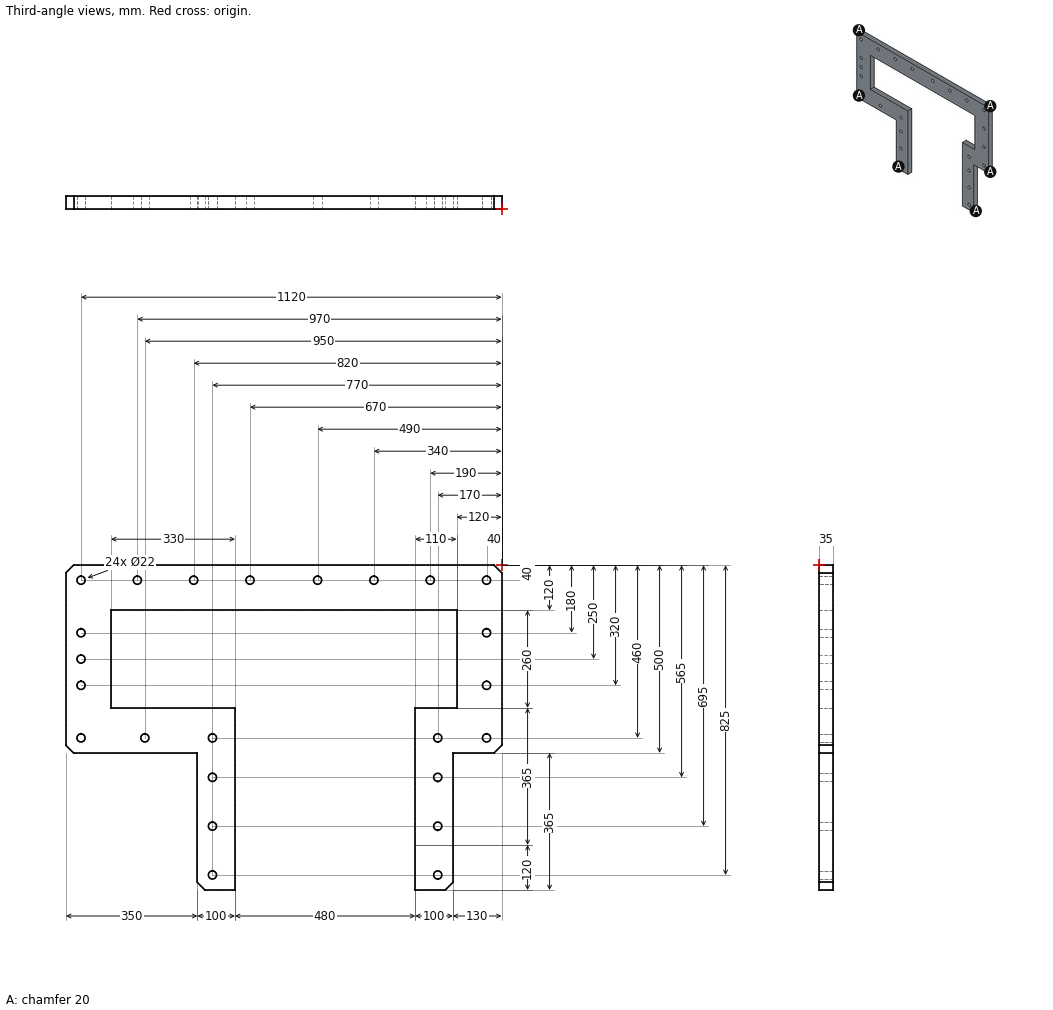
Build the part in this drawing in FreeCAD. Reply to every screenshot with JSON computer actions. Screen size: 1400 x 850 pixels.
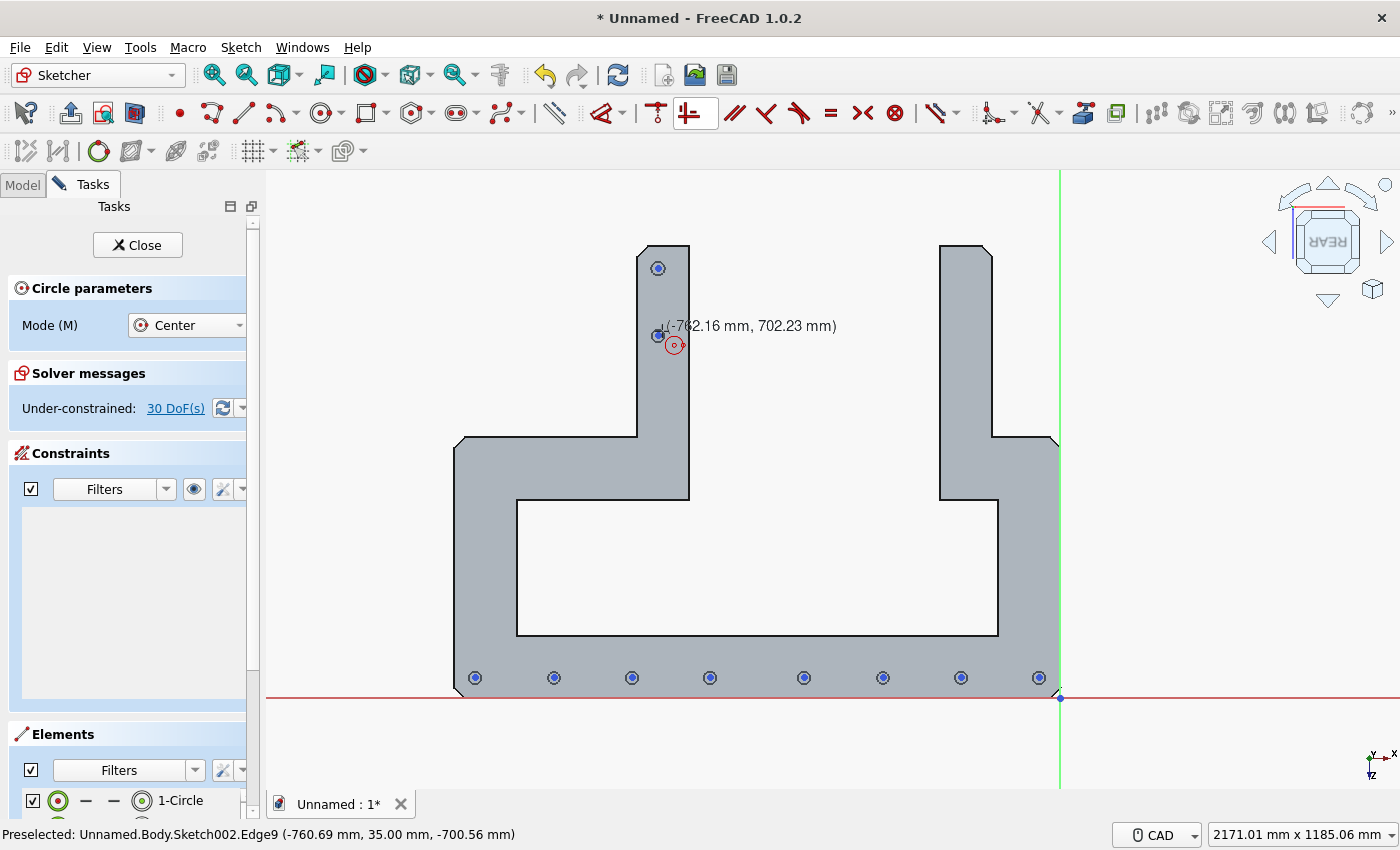
{"action": "left_click", "coordinate": [658, 403]}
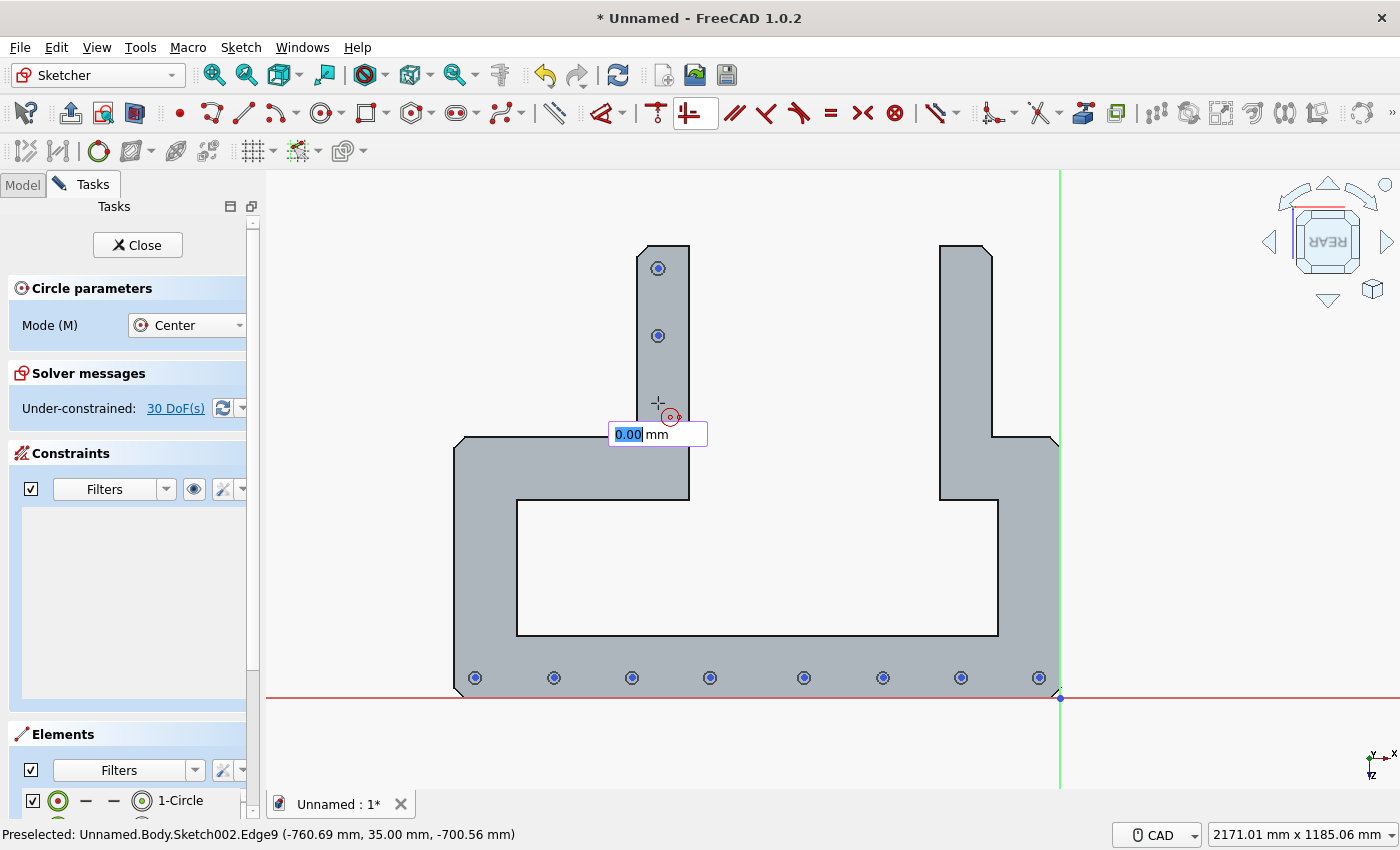
{"action": "scroll", "coordinate": [662, 399], "scroll_direction": "up", "scroll_amount": 6}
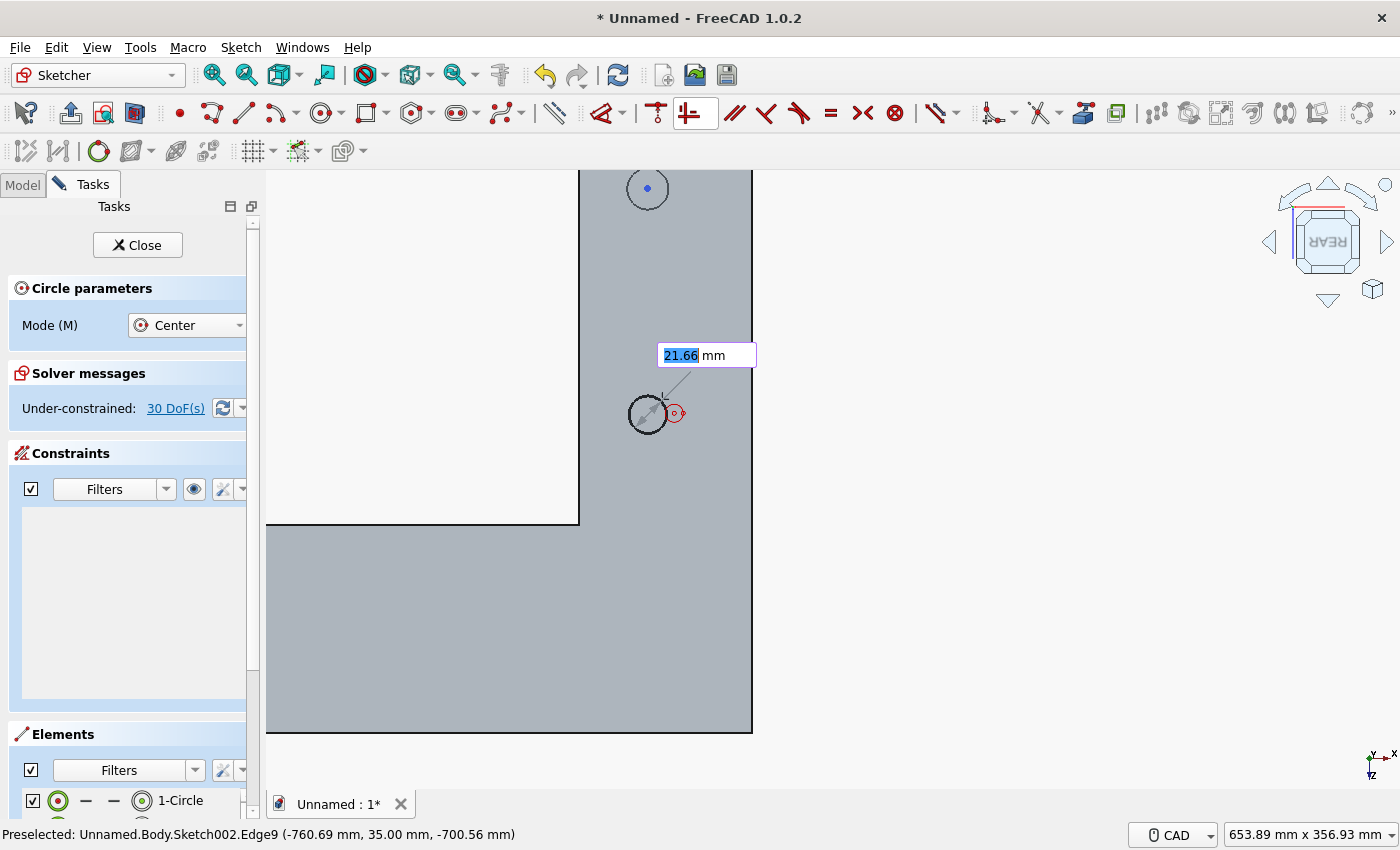
{"action": "left_click", "coordinate": [662, 398]}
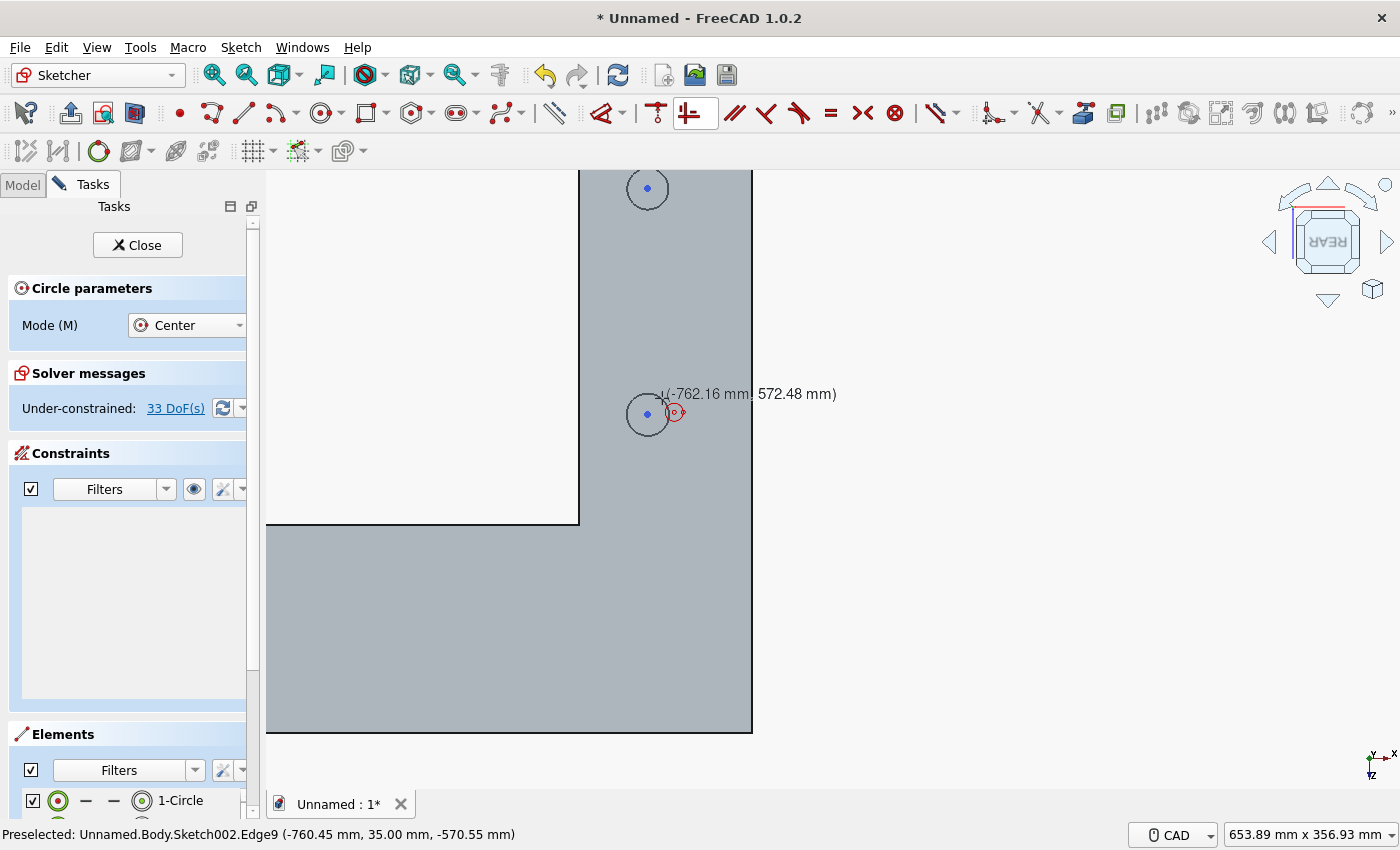
{"action": "scroll", "coordinate": [662, 399], "scroll_direction": "down", "scroll_amount": 6}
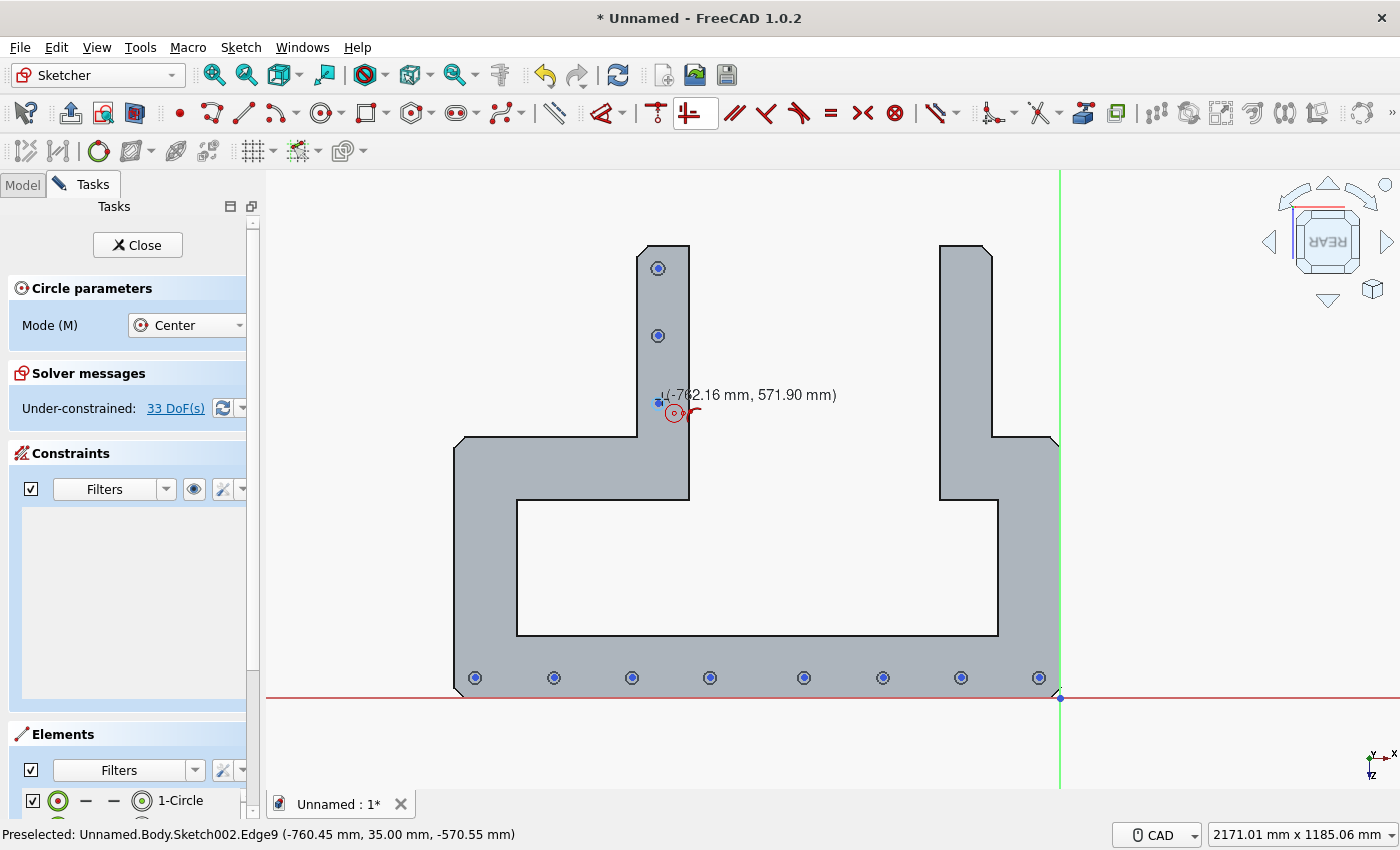
{"action": "left_click", "coordinate": [658, 458]}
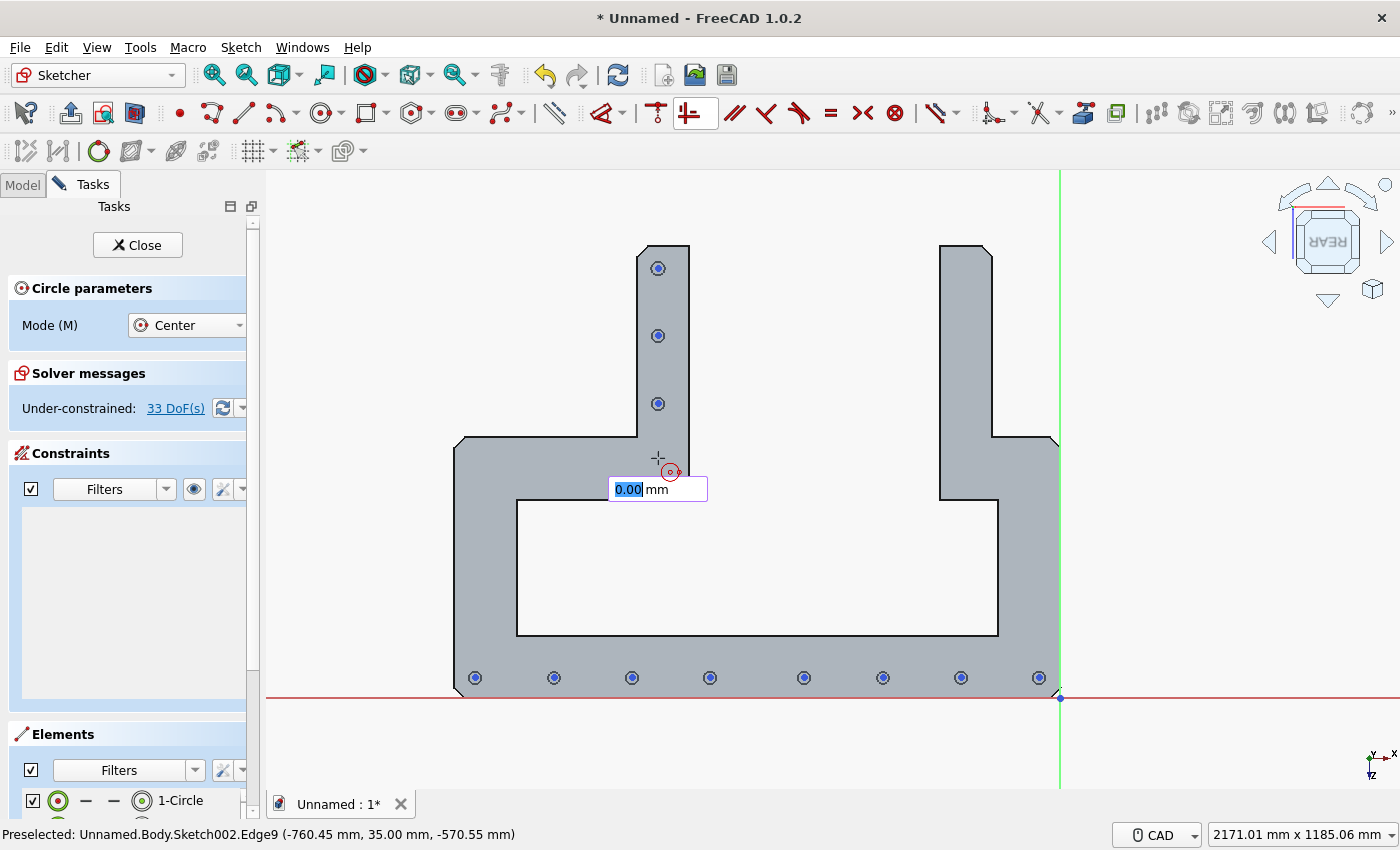
{"action": "scroll", "coordinate": [662, 454], "scroll_direction": "up", "scroll_amount": 6}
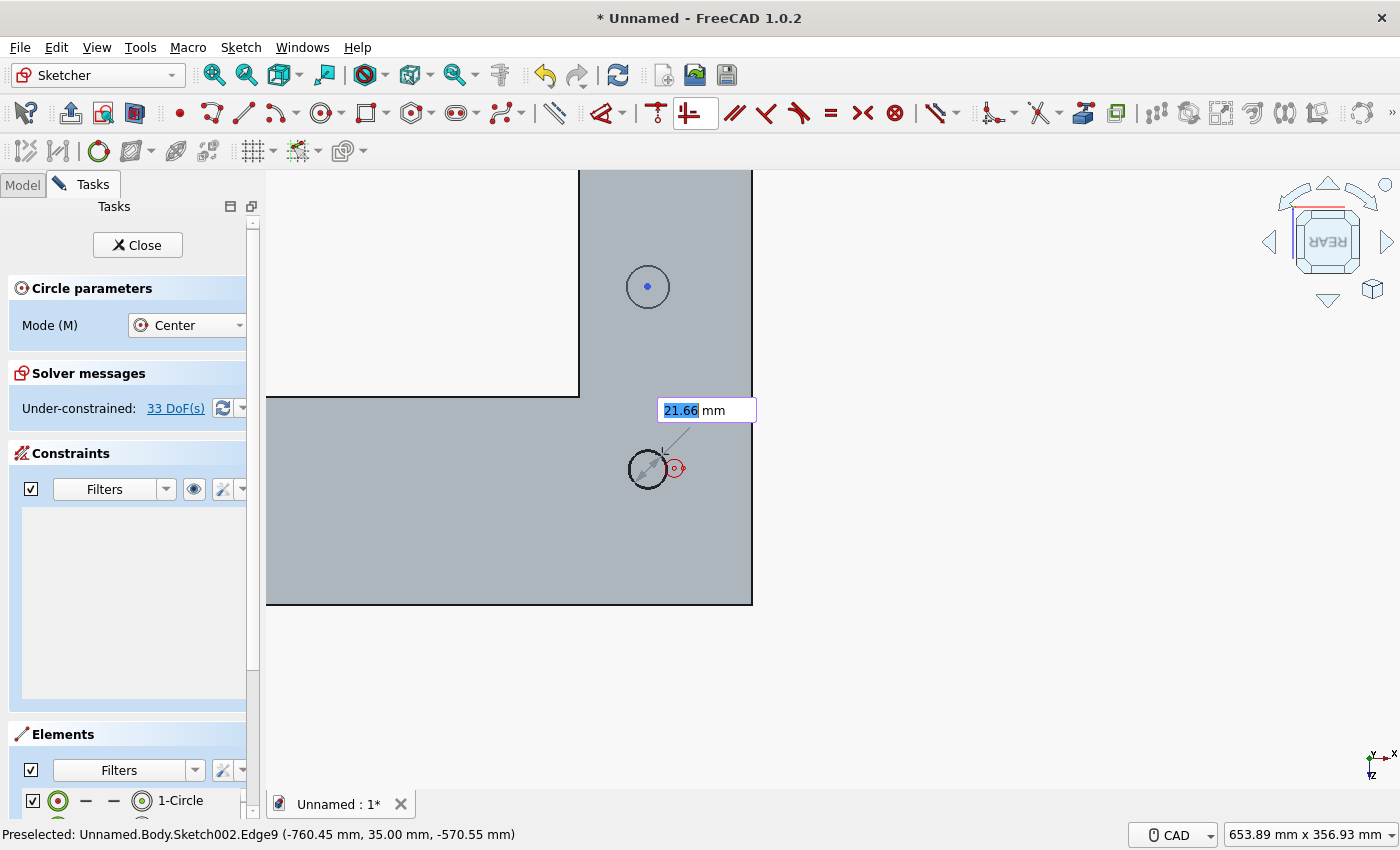
{"action": "left_click", "coordinate": [662, 453]}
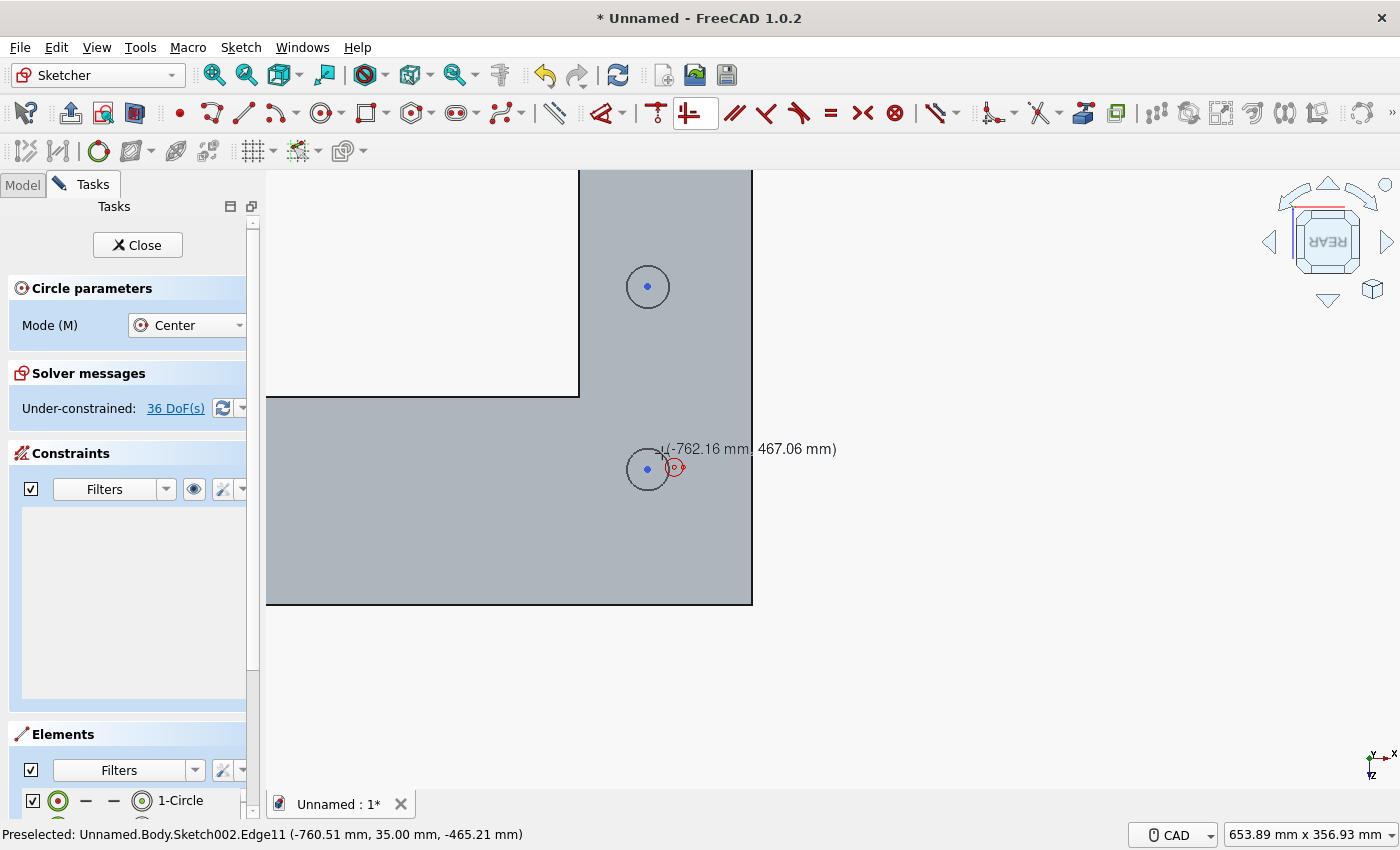
{"action": "scroll", "coordinate": [662, 454], "scroll_direction": "down", "scroll_amount": 6}